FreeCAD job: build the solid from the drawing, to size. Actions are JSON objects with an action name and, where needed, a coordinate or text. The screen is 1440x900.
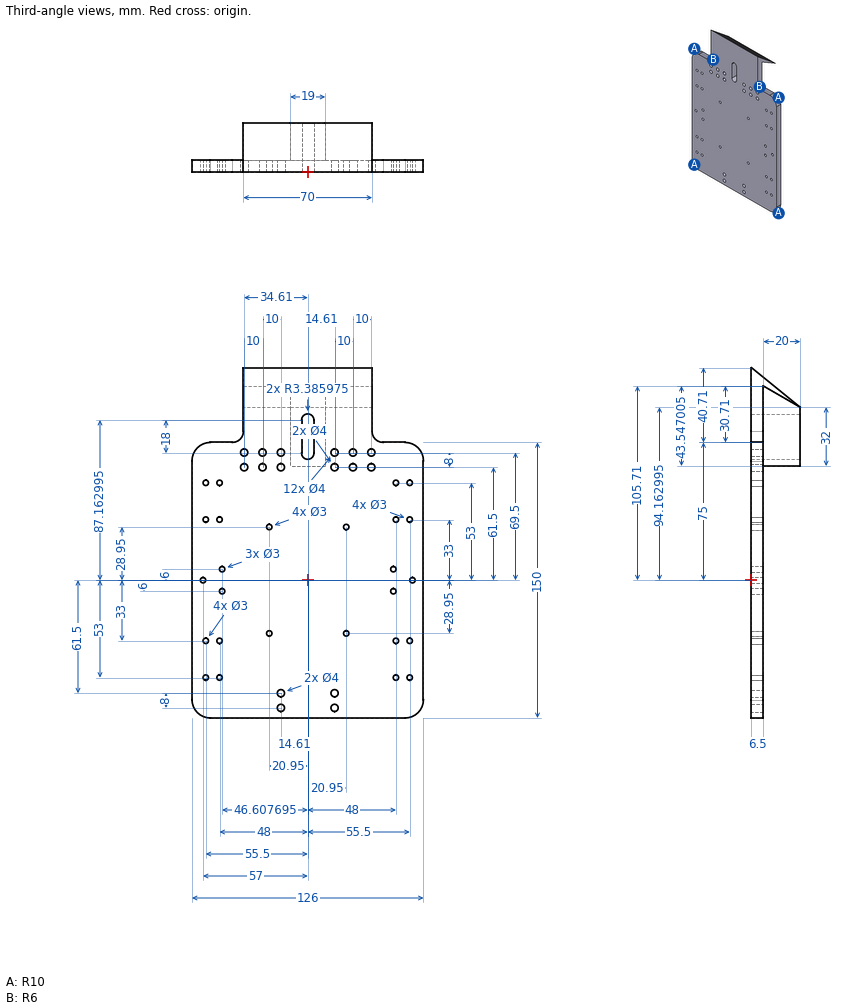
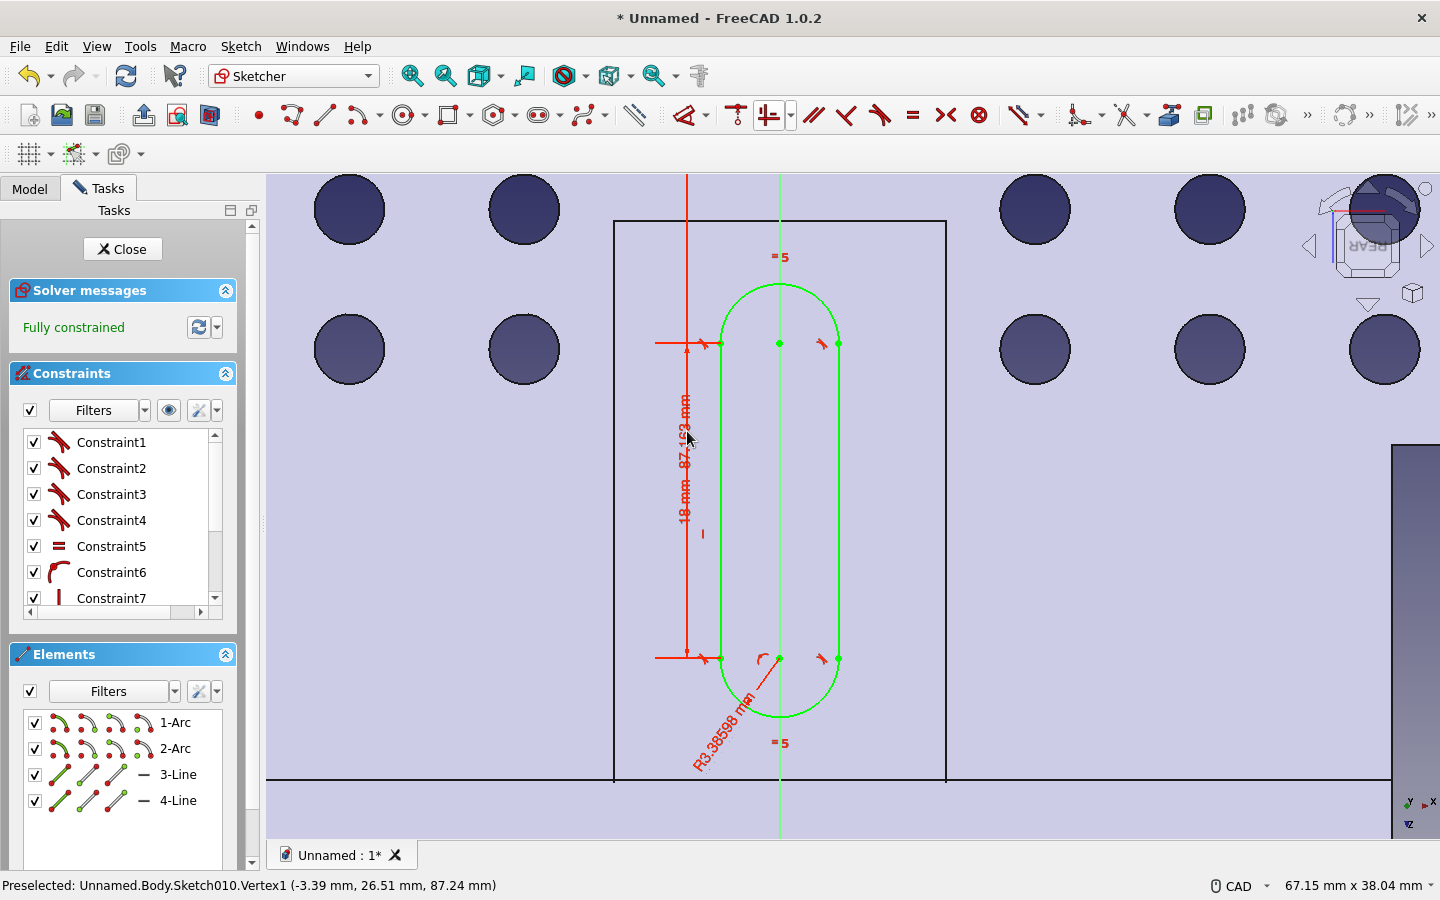
{"action": "left_click", "coordinate": [123, 249]}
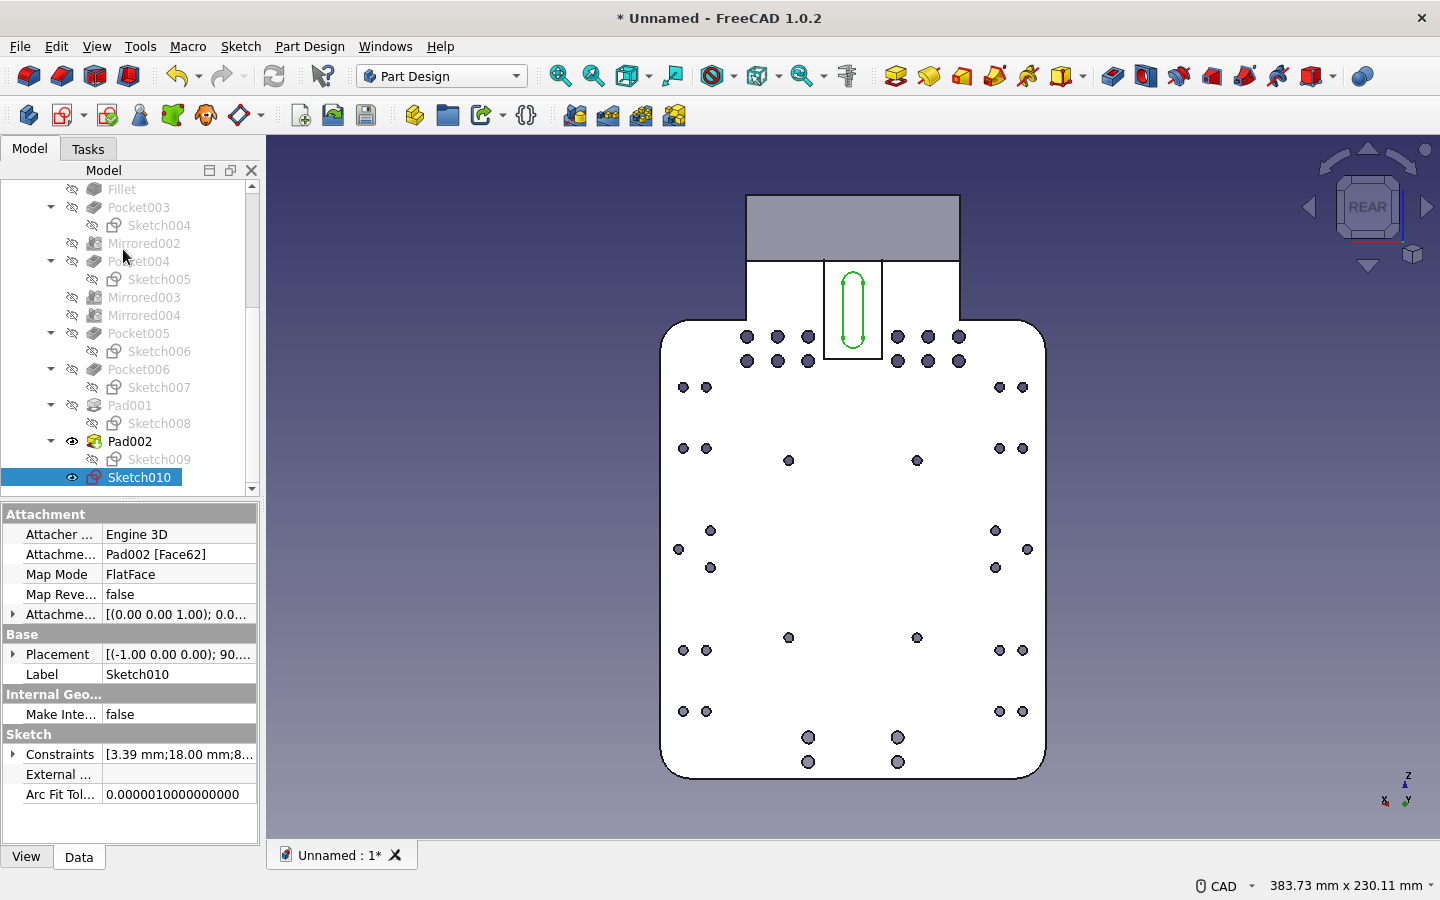
{"action": "left_click", "coordinate": [1113, 76]}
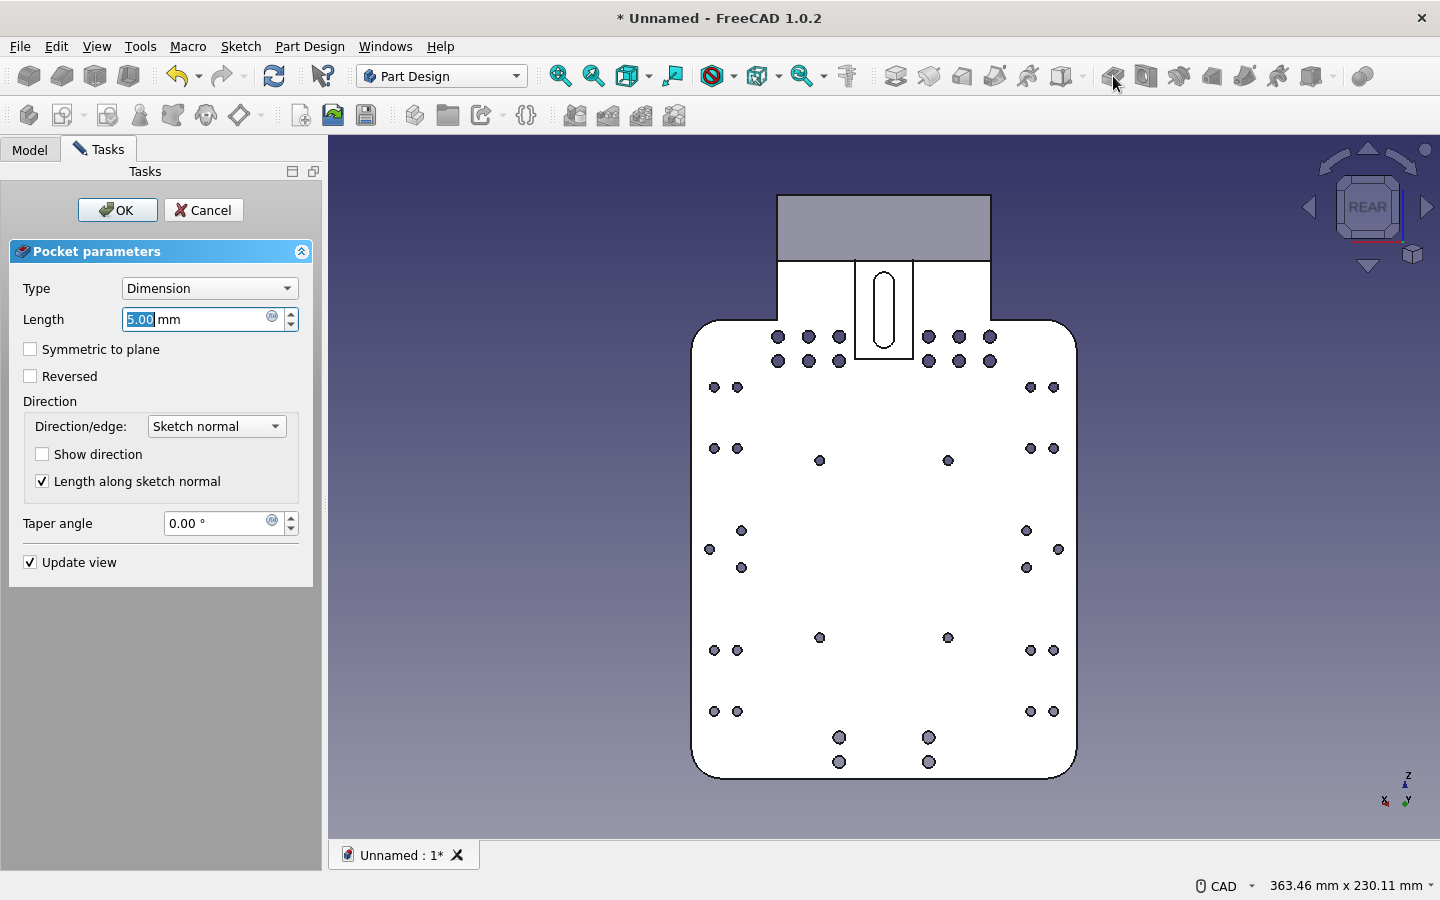
{"action": "left_click", "coordinate": [210, 288]}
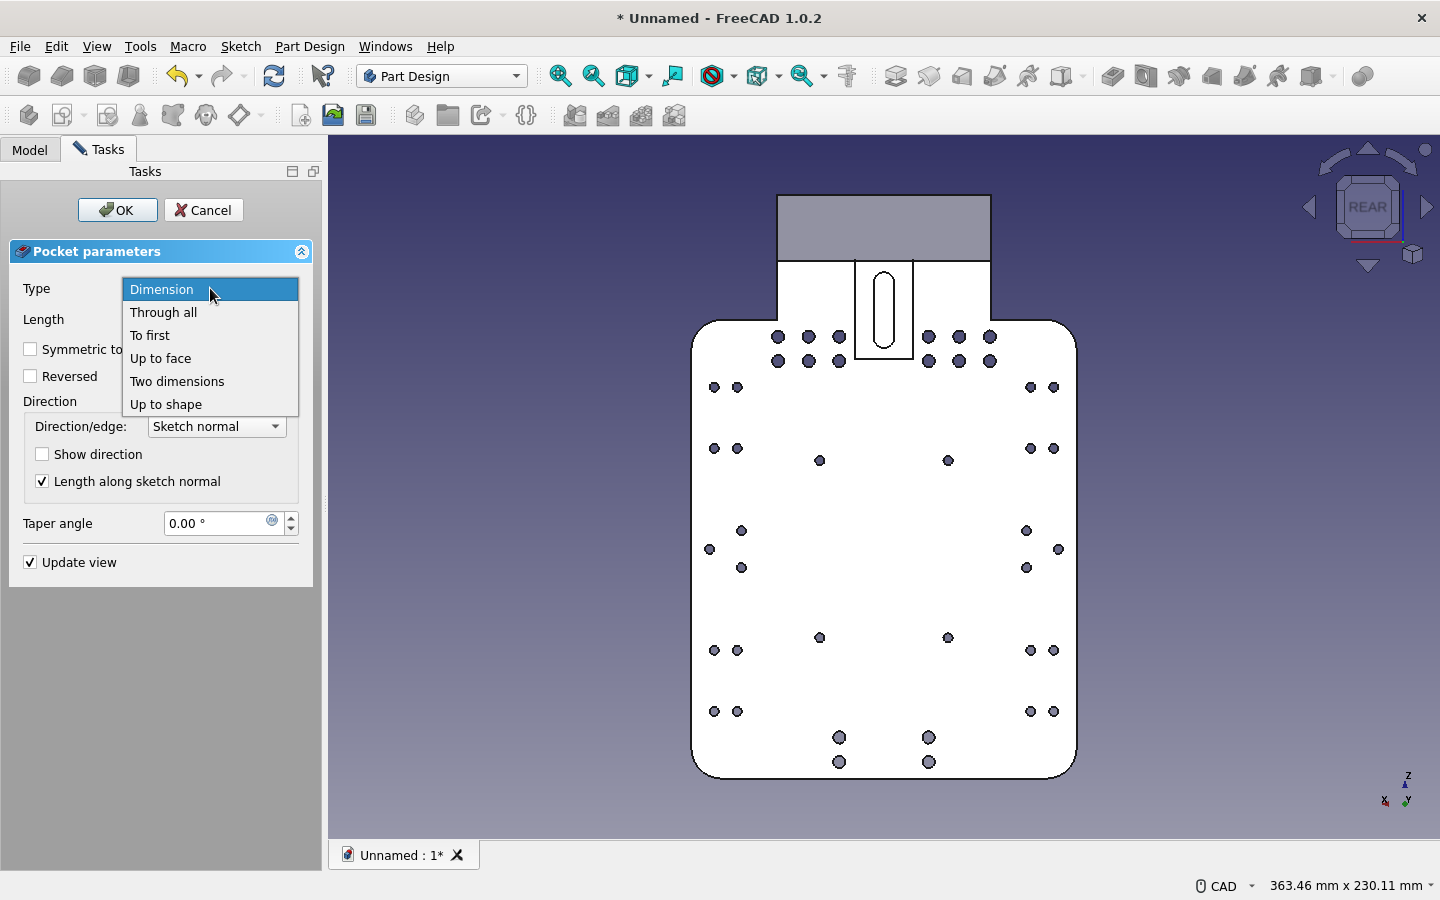
{"action": "left_click", "coordinate": [208, 312]}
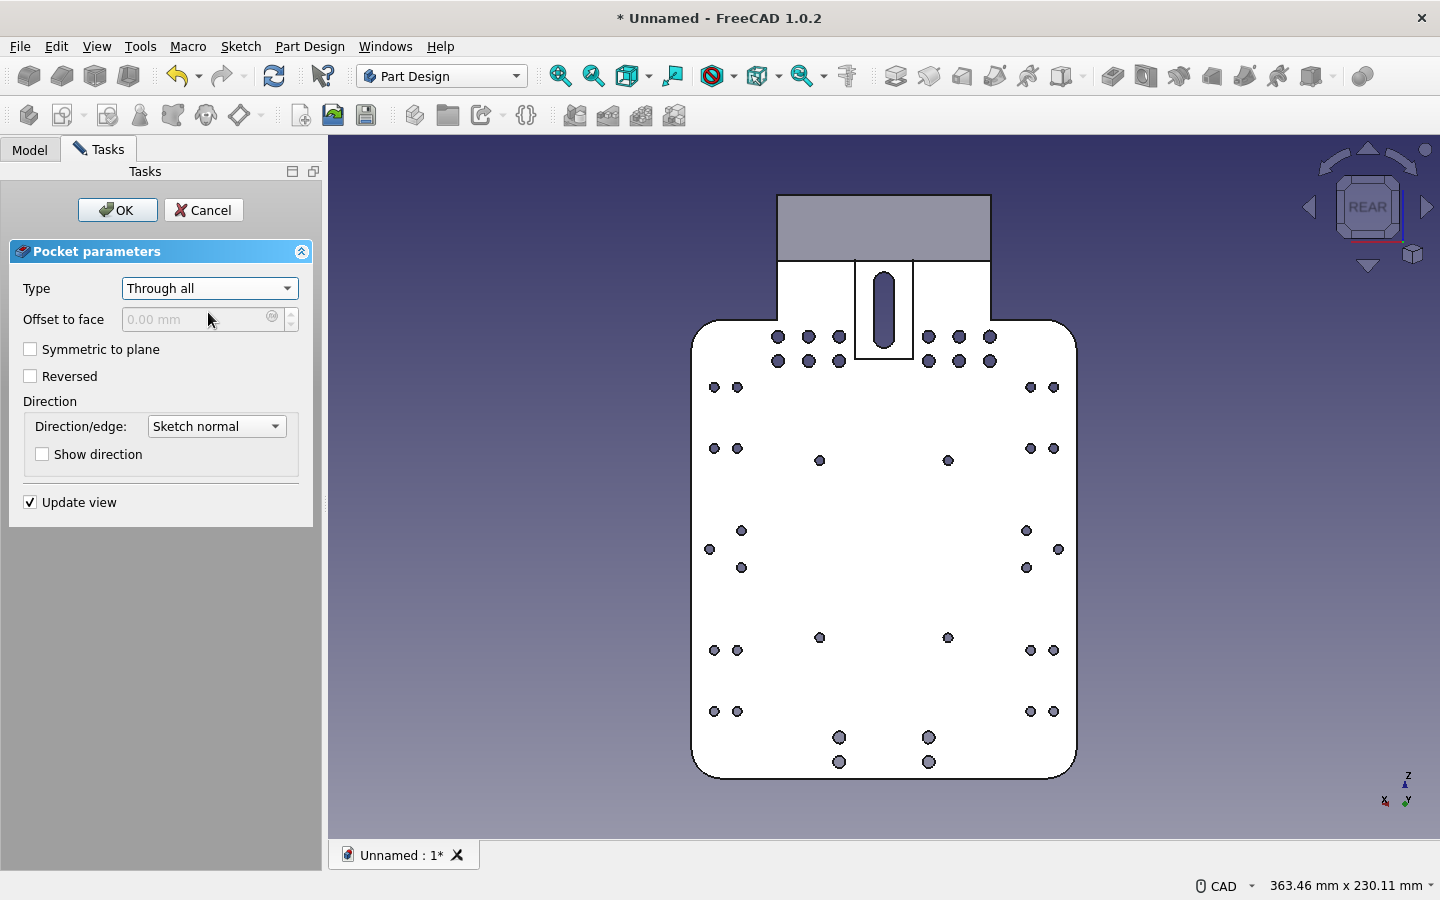
{"action": "left_click", "coordinate": [118, 210]}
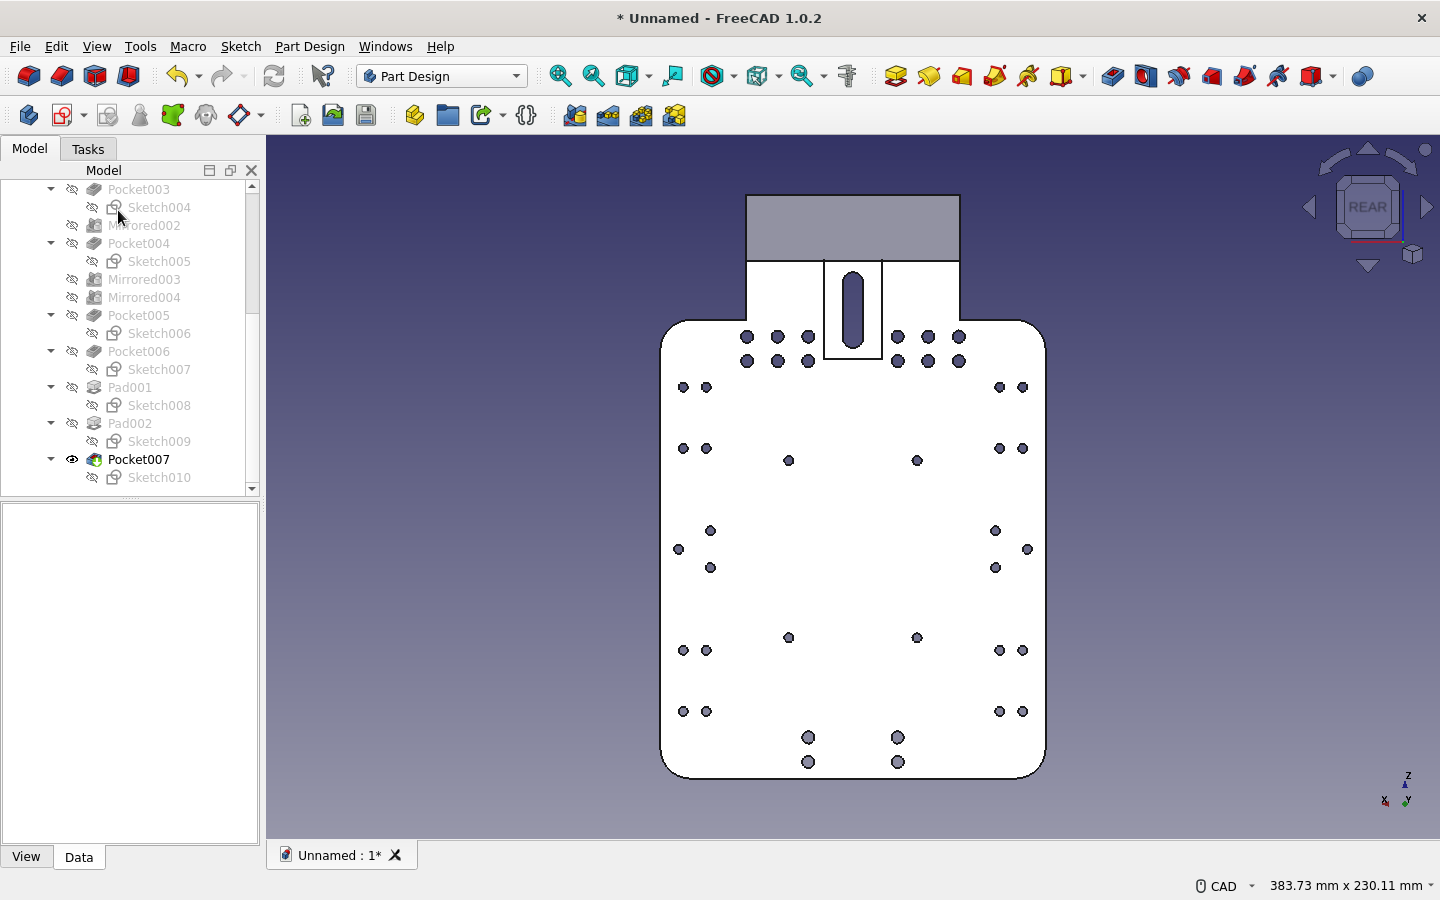
{"action": "scroll", "coordinate": [960, 319], "scroll_direction": "up", "scroll_amount": 4}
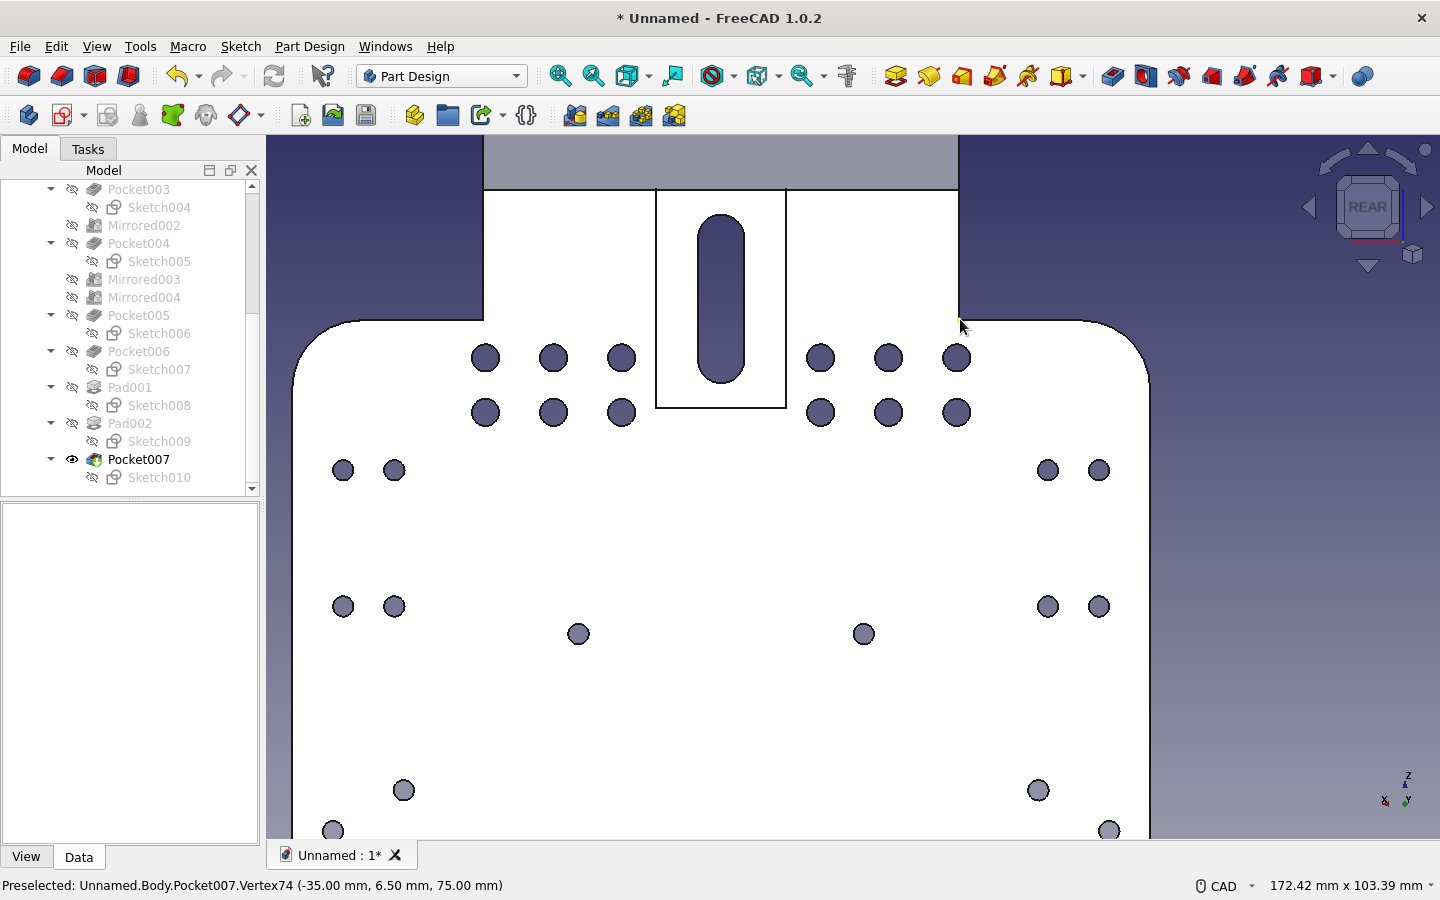
{"action": "left_click", "coordinate": [561, 76]}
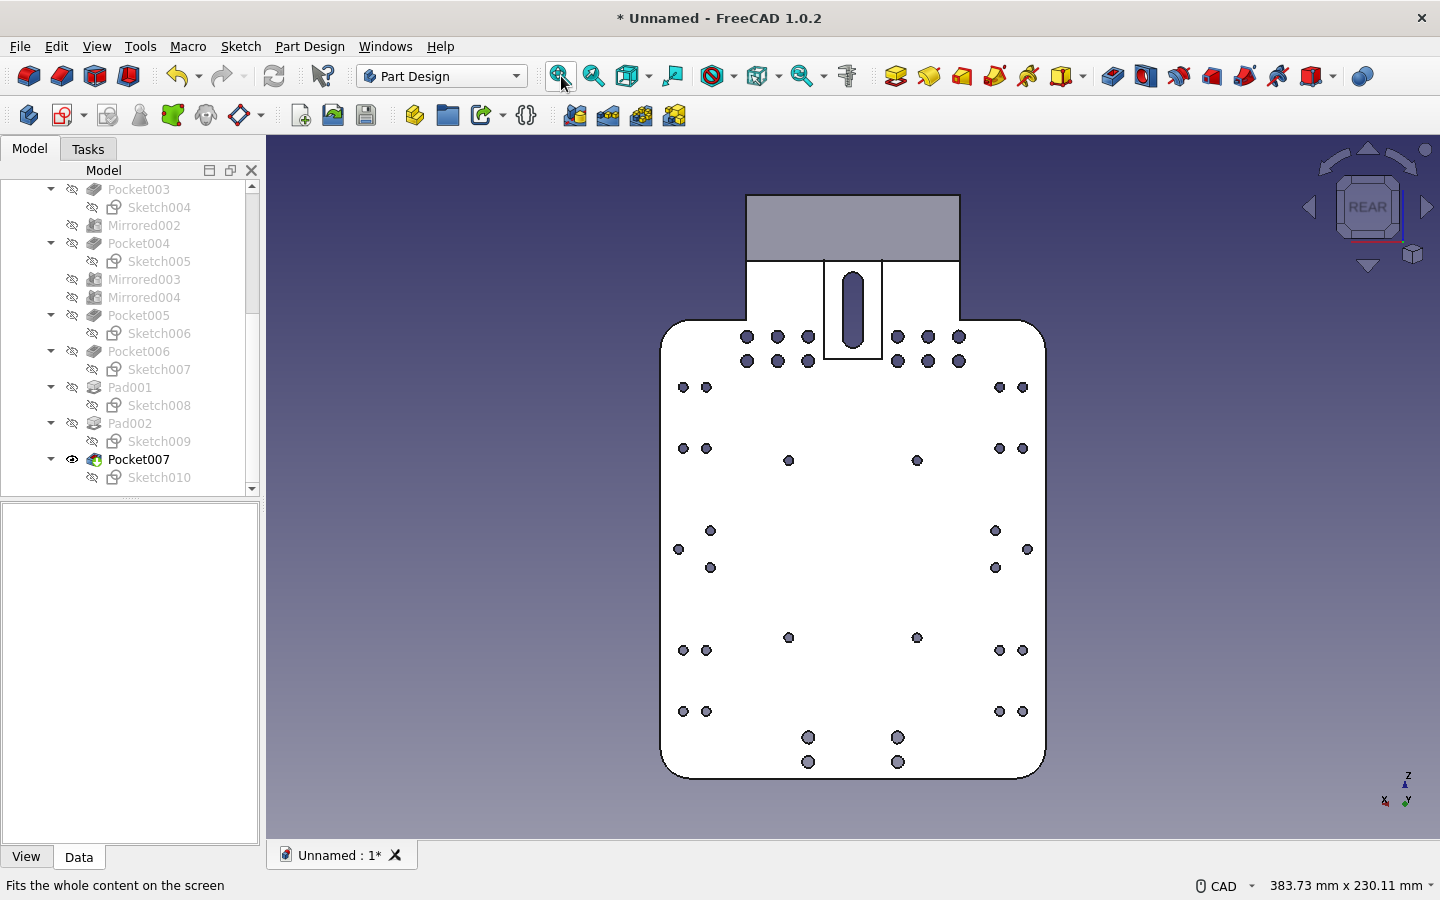
{"action": "key", "text": "0"}